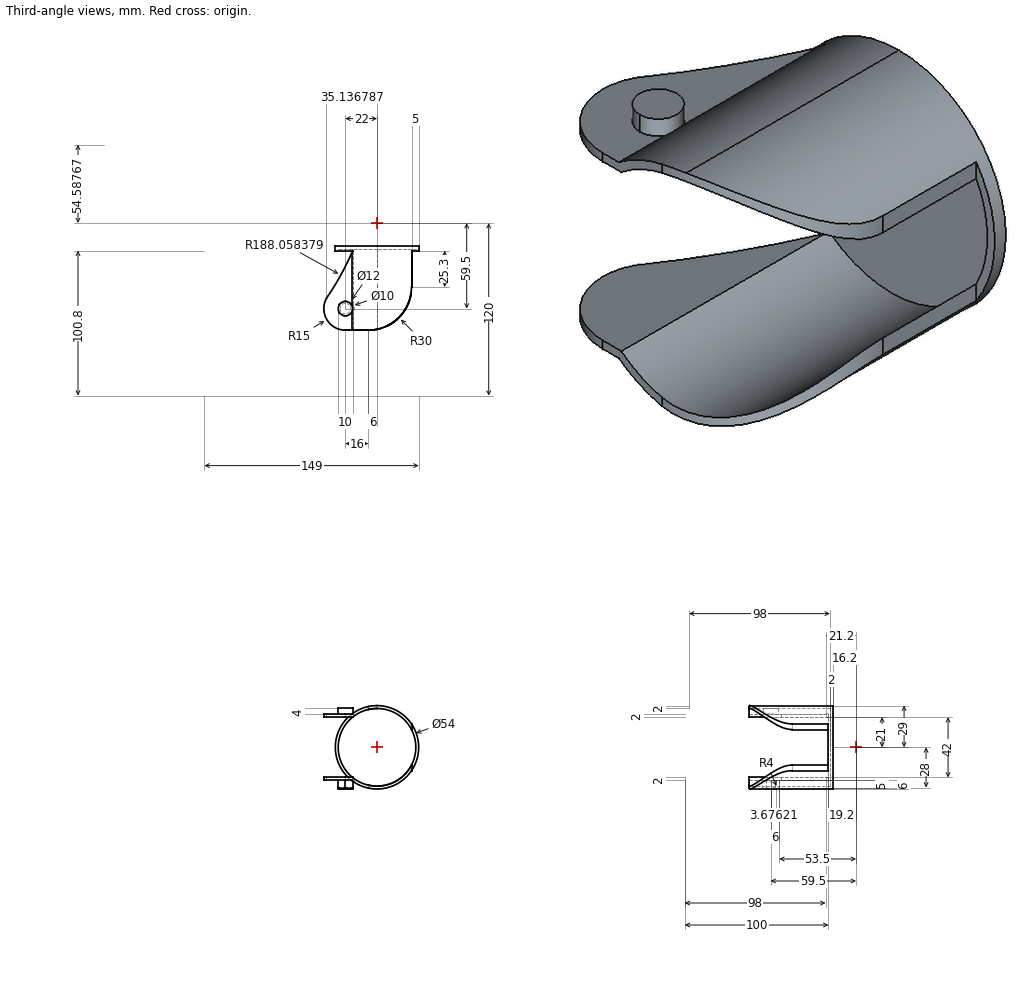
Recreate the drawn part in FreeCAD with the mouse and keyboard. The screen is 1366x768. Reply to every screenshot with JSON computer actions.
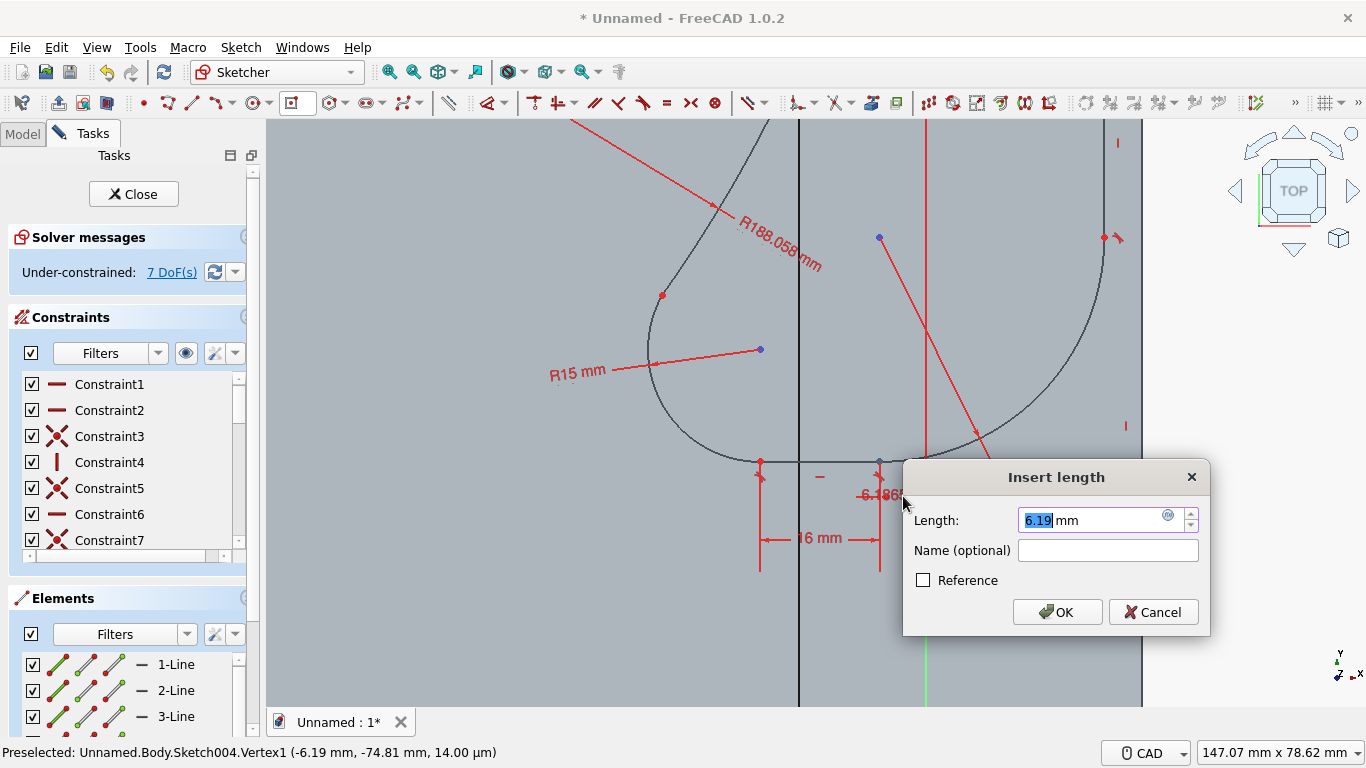
{"action": "type", "text": "6"}
{"action": "key", "text": "Return"}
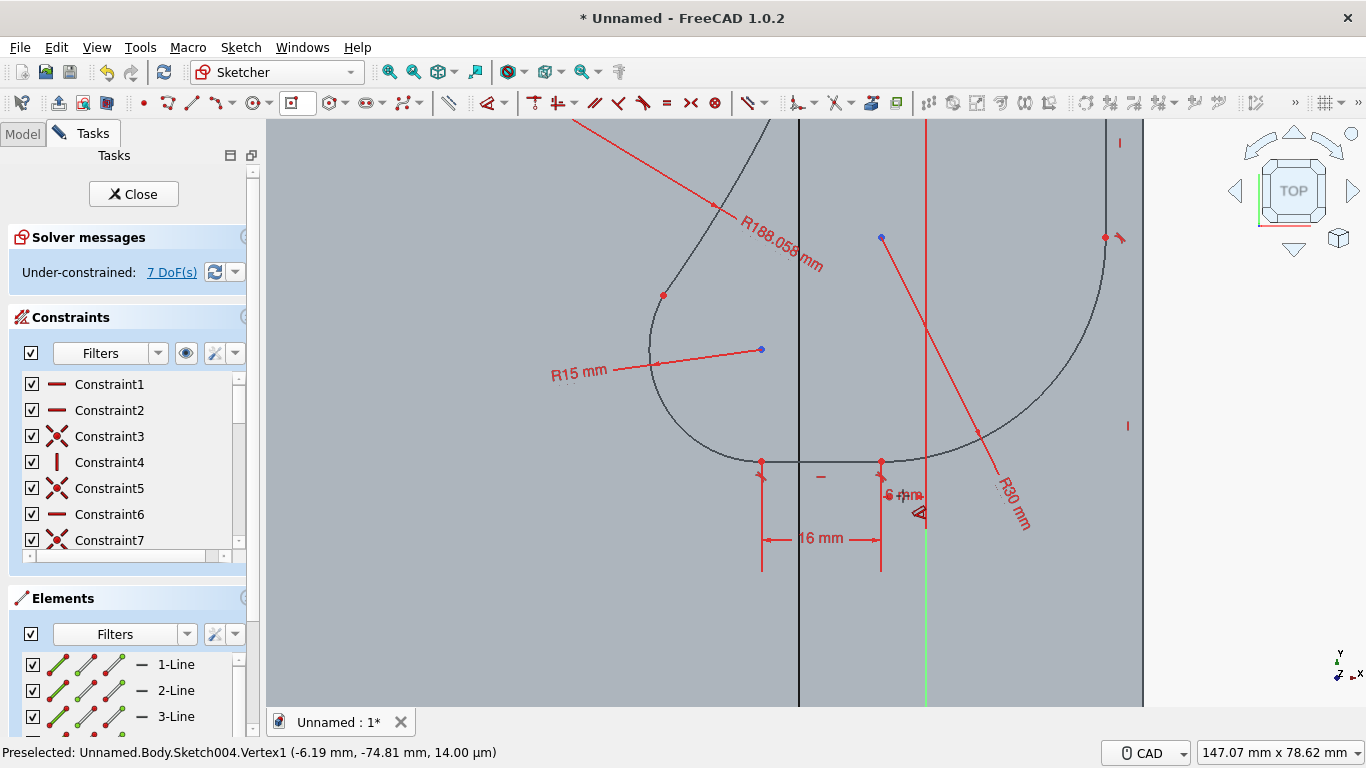
{"action": "scroll", "coordinate": [879, 464], "scroll_direction": "down", "scroll_amount": 4}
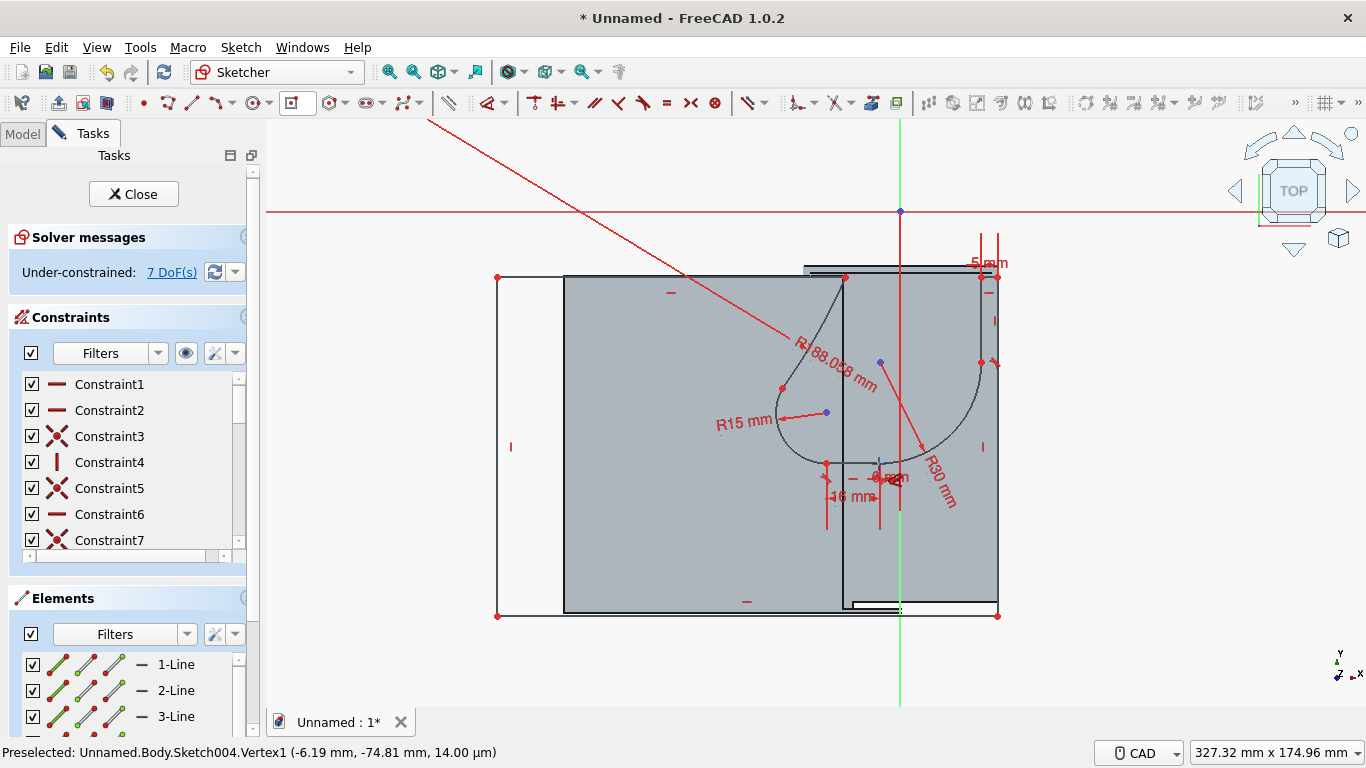
{"action": "left_click", "coordinate": [647, 616]}
{"action": "left_click", "coordinate": [748, 650]}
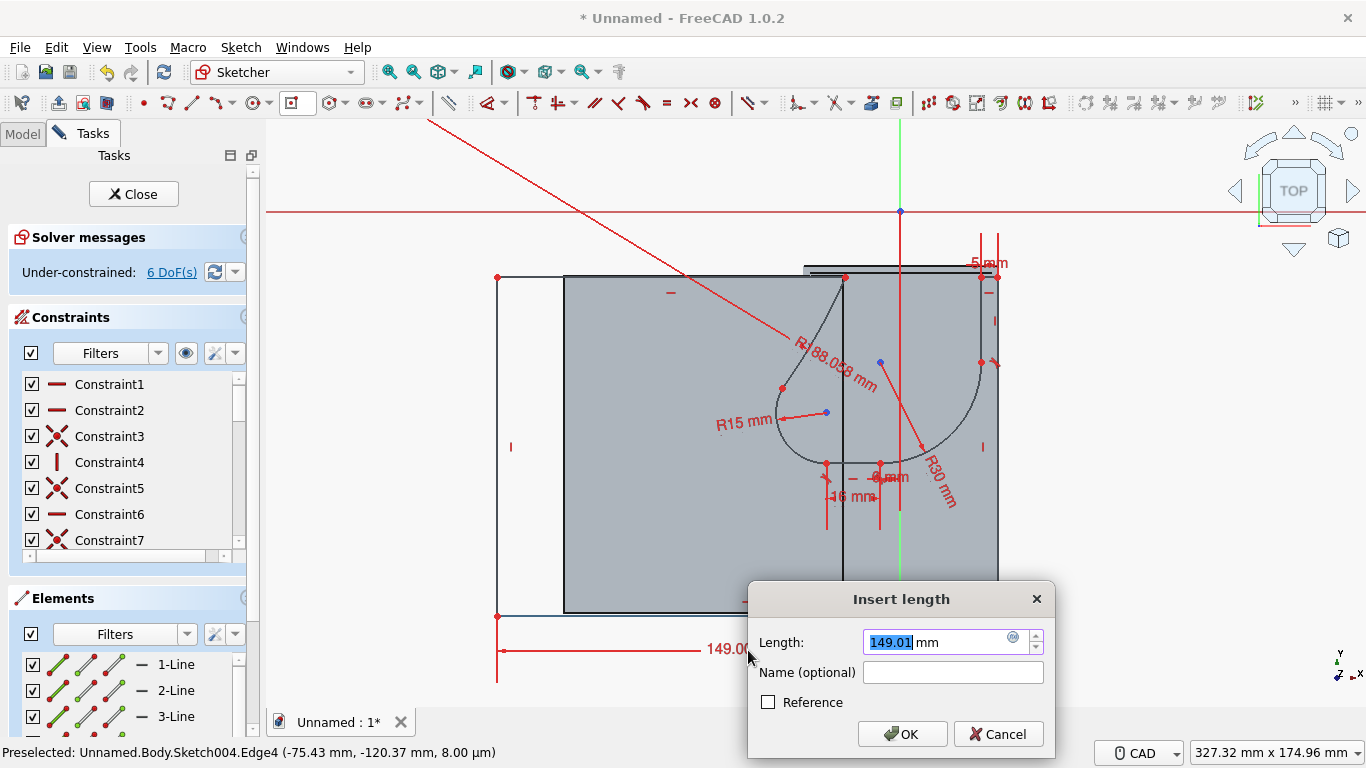
{"action": "type", "text": "149"}
{"action": "key", "text": "Return"}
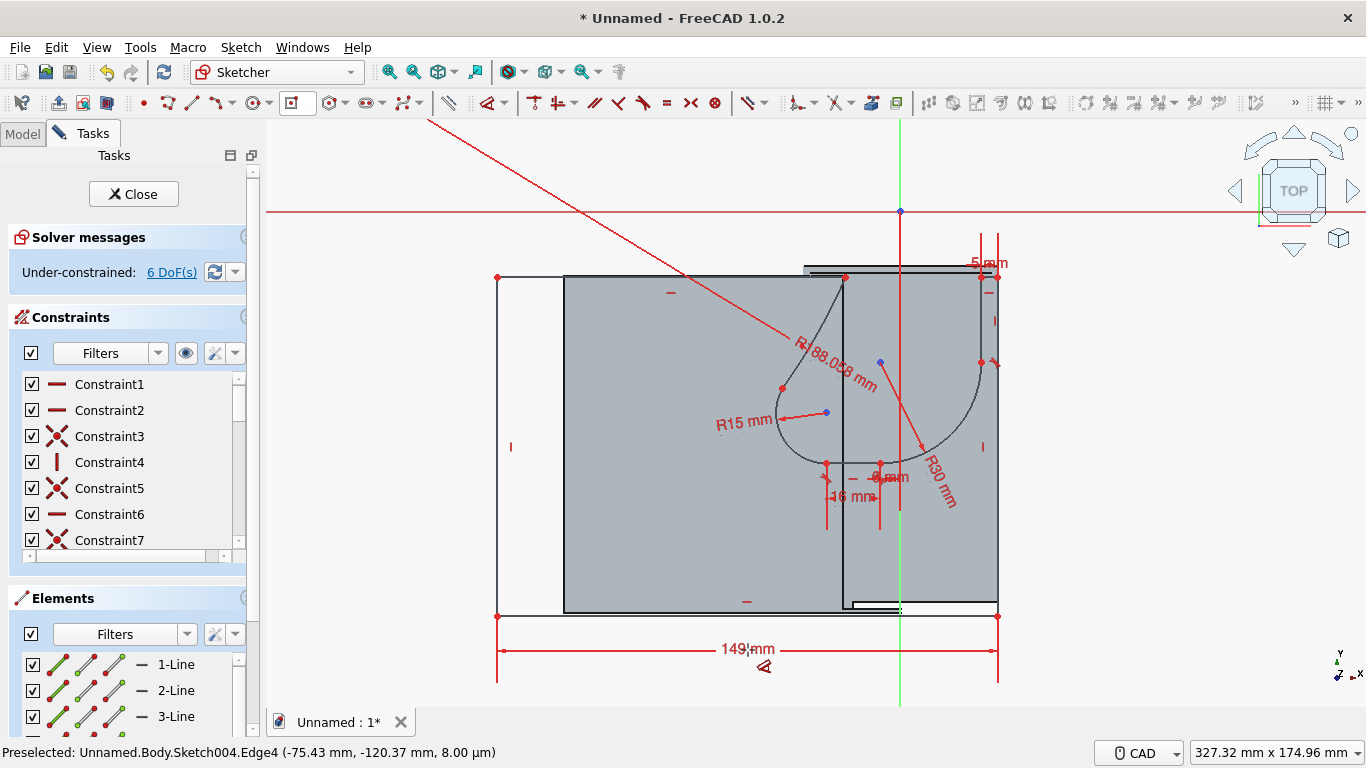
{"action": "left_click", "coordinate": [981, 303]}
{"action": "left_click", "coordinate": [1015, 320]}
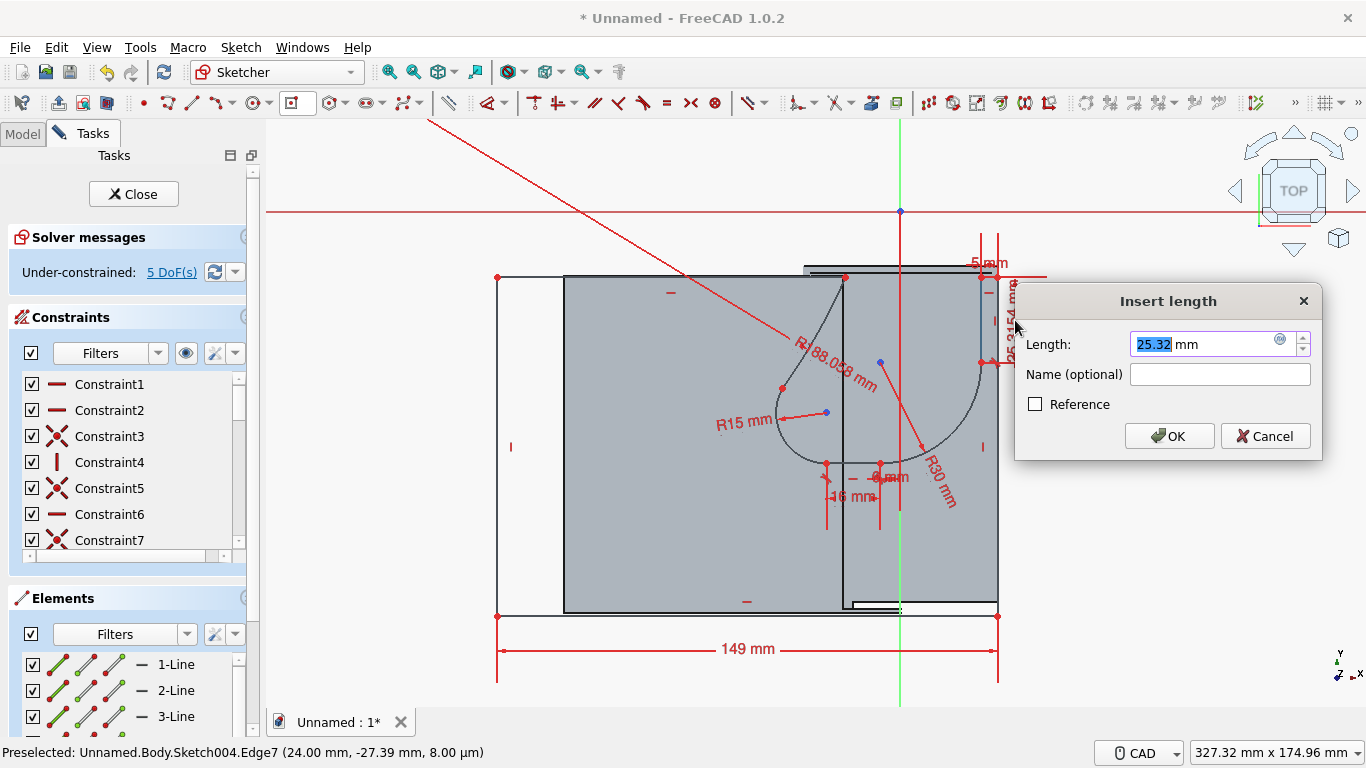
{"action": "type", "text": "25.3"}
{"action": "key", "text": "Return"}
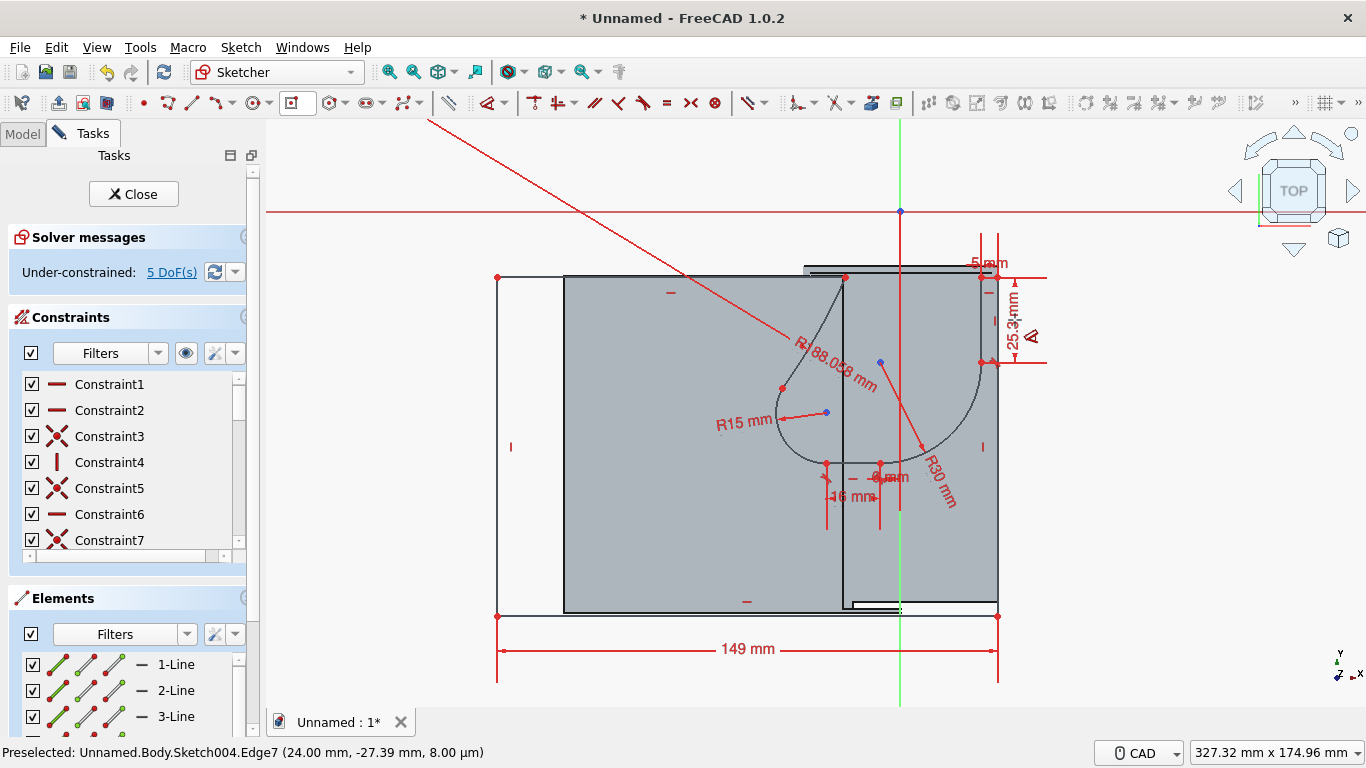
{"action": "left_click", "coordinate": [497, 616]}
{"action": "left_click", "coordinate": [463, 414]}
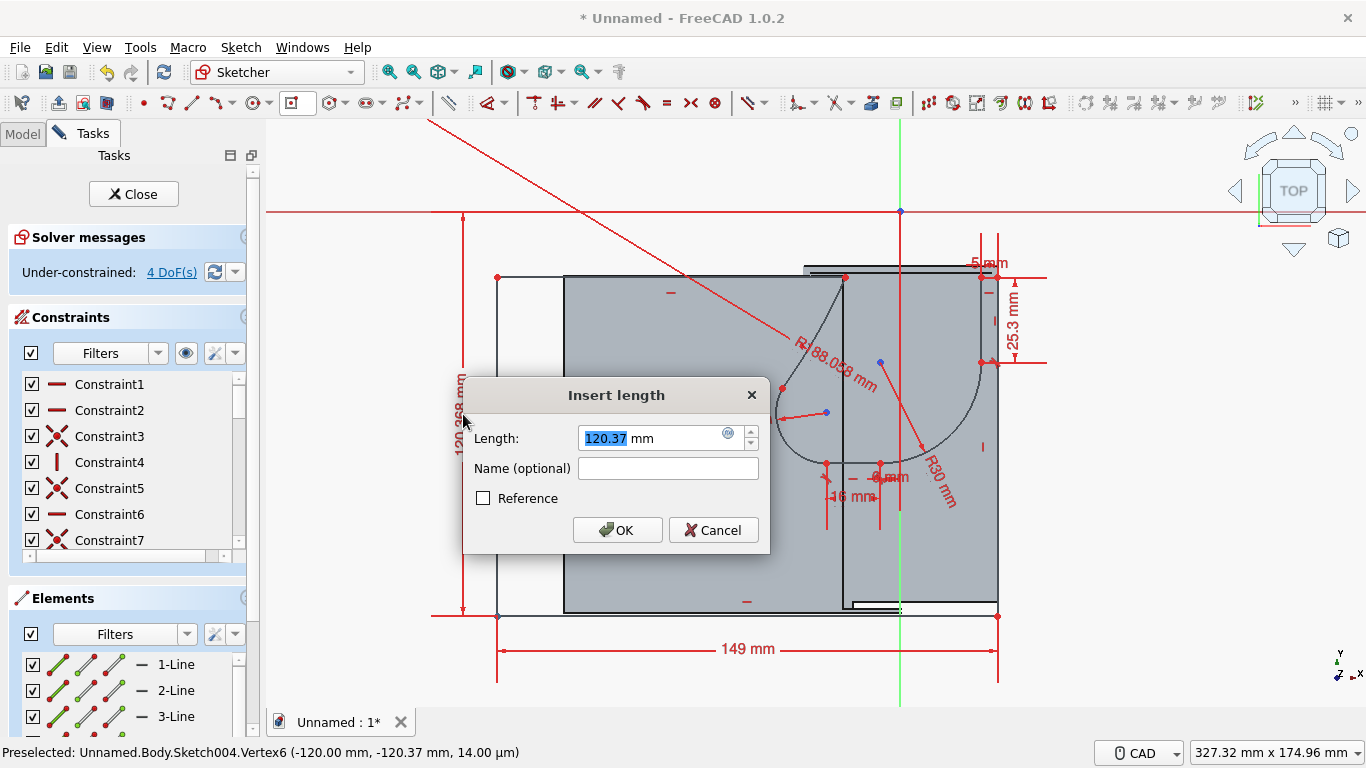
{"action": "type", "text": "120"}
{"action": "key", "text": "Return"}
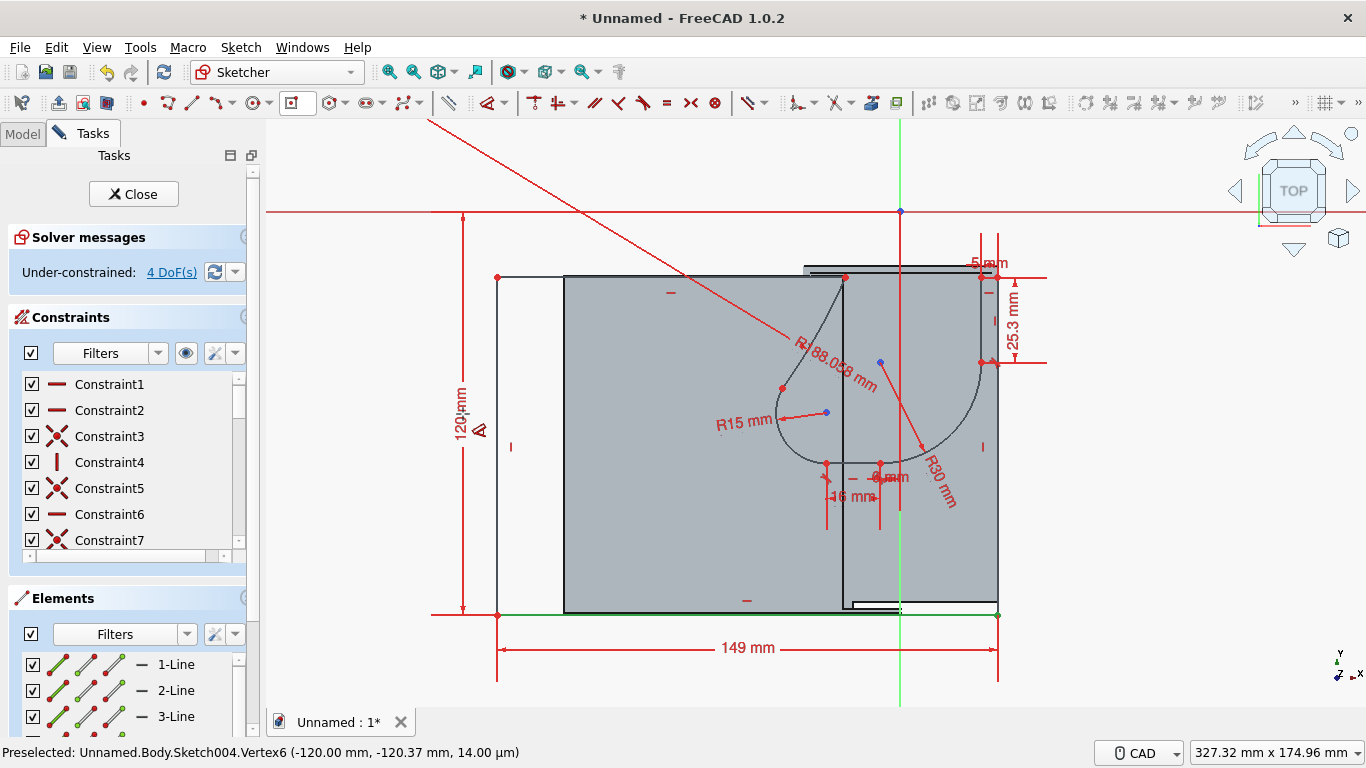
{"action": "left_click", "coordinate": [497, 379]}
{"action": "left_click", "coordinate": [463, 446]}